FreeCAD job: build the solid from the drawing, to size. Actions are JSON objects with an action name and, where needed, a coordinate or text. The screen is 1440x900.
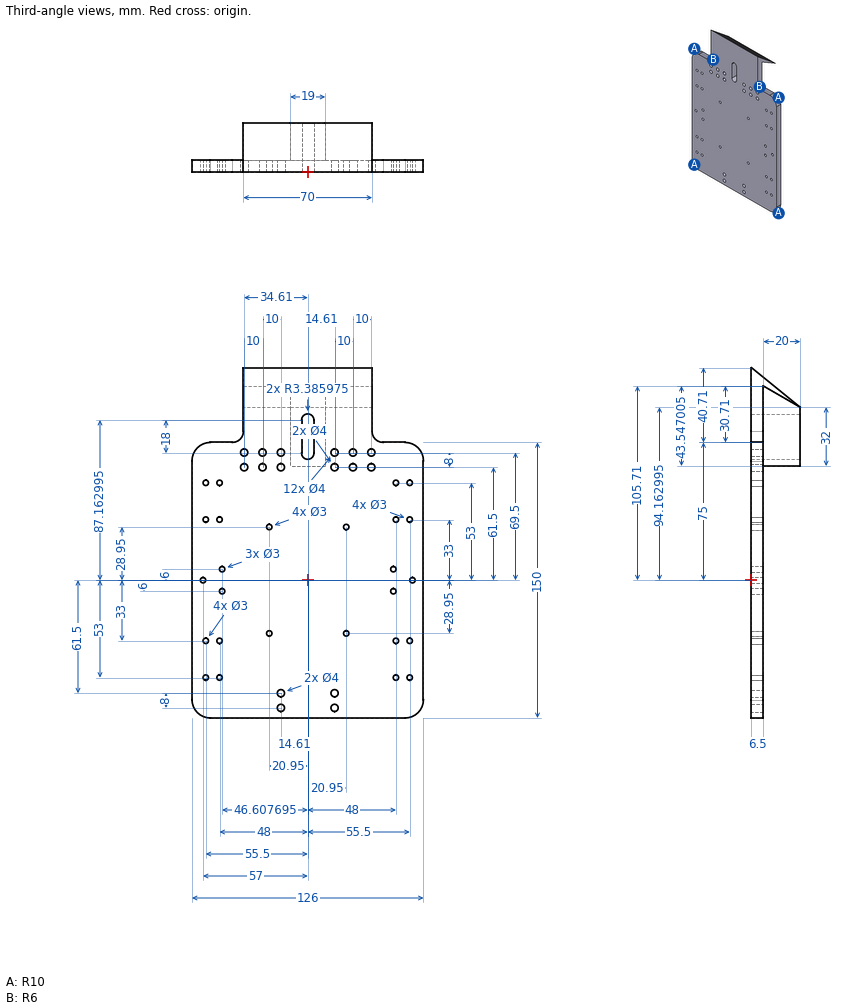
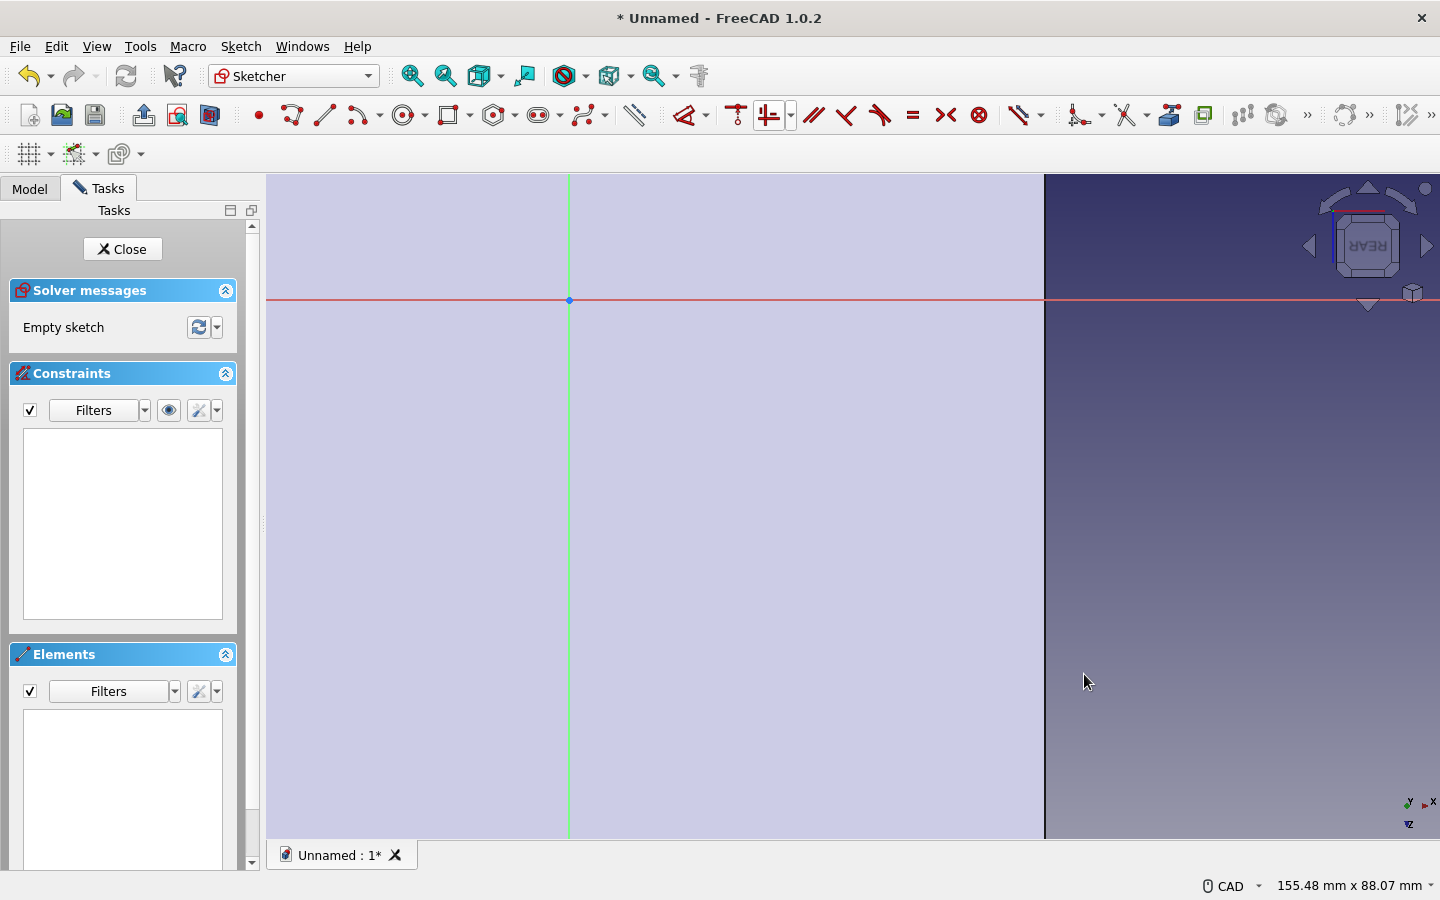
{"action": "key", "text": "g c"}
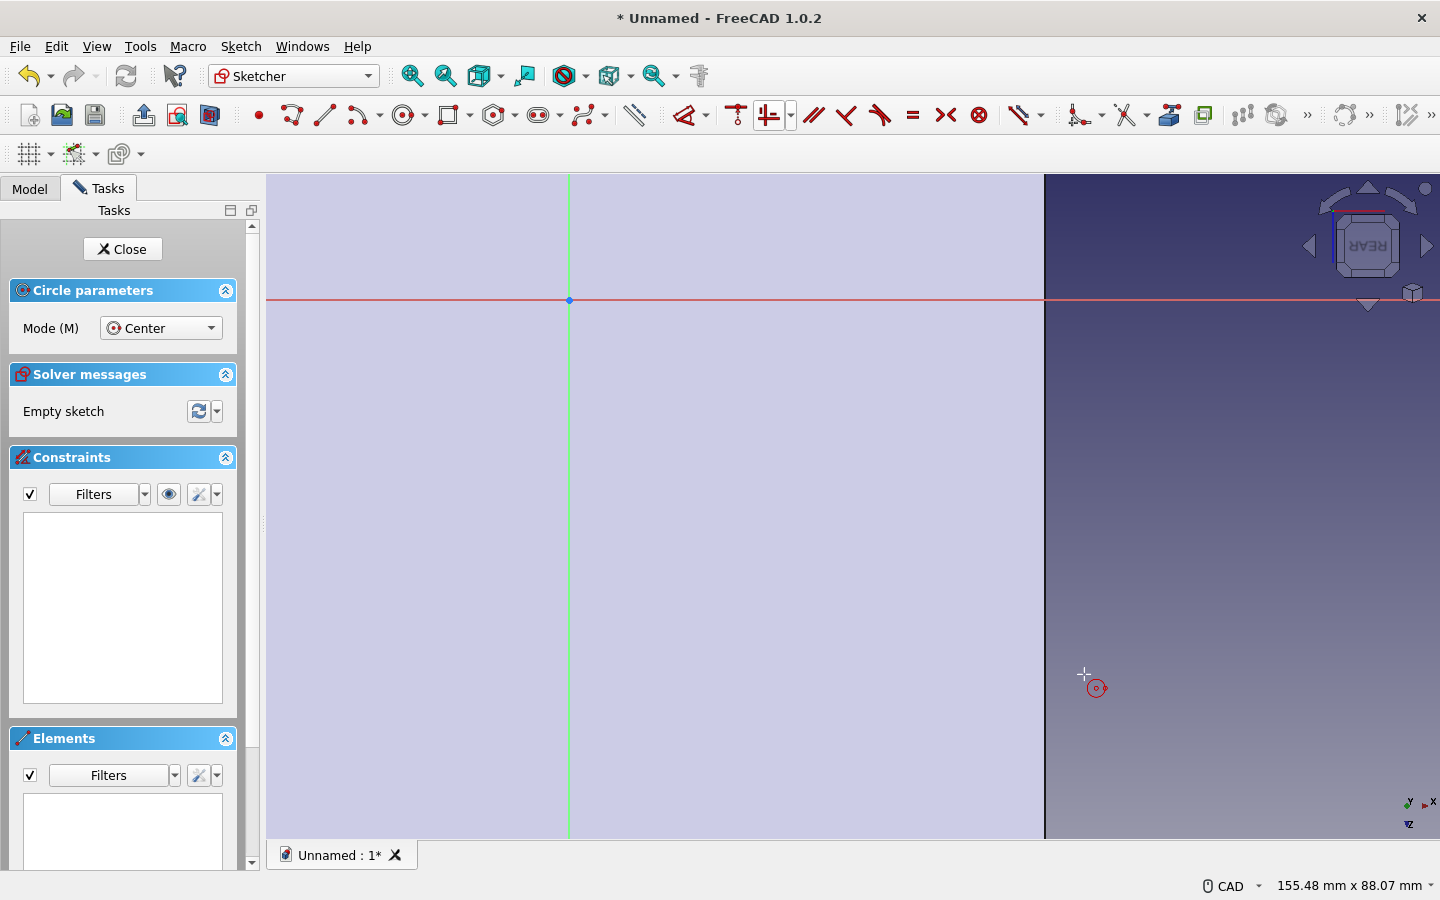
{"action": "scroll", "coordinate": [988, 549], "scroll_direction": "up", "scroll_amount": 4}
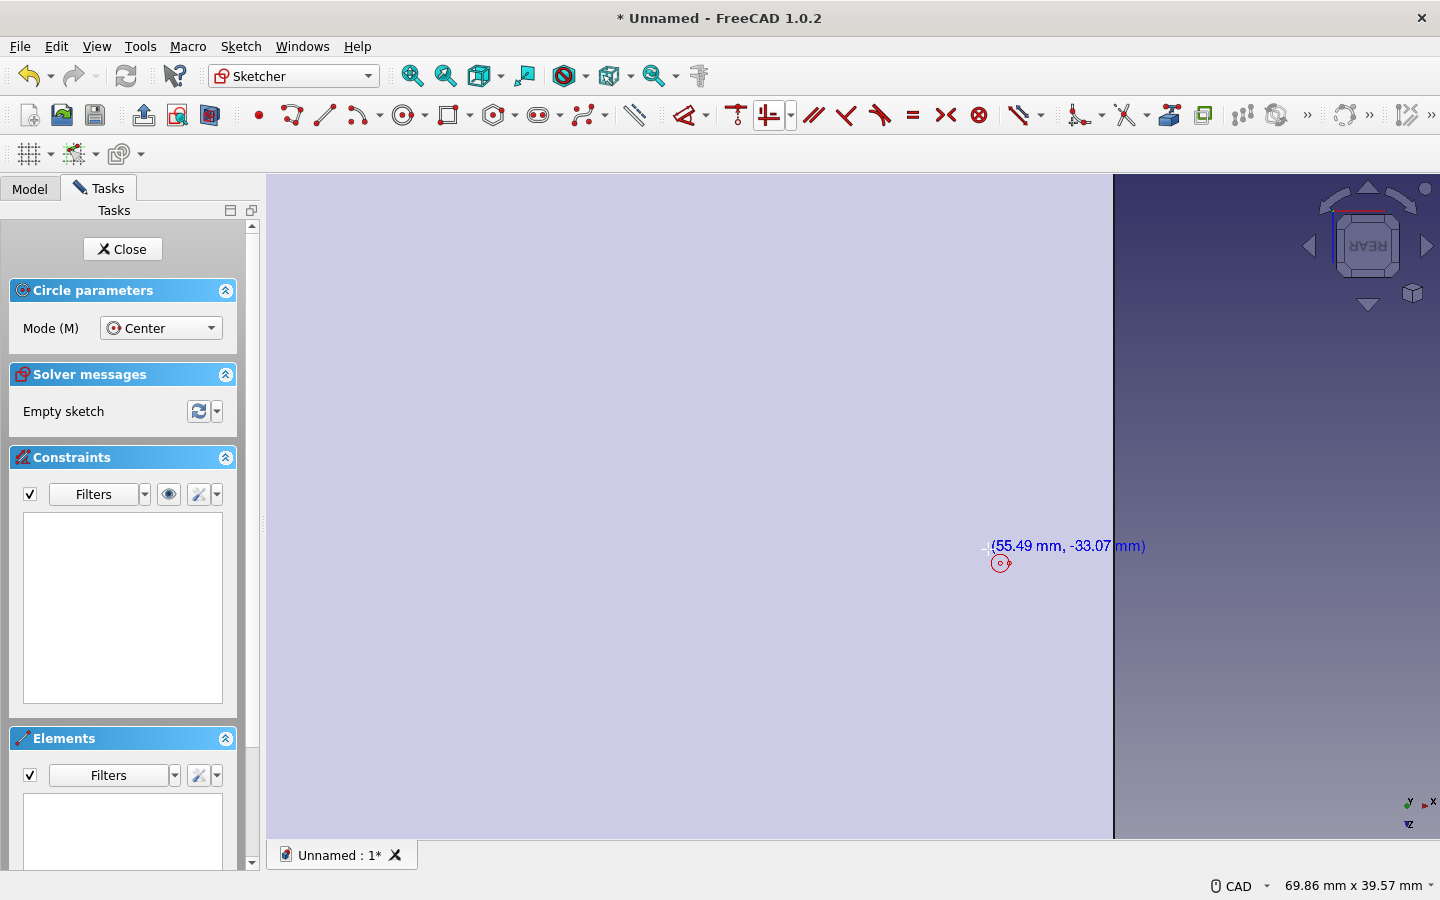
{"action": "left_click", "coordinate": [987, 549]}
{"action": "mouse_move", "coordinate": [1005, 532]}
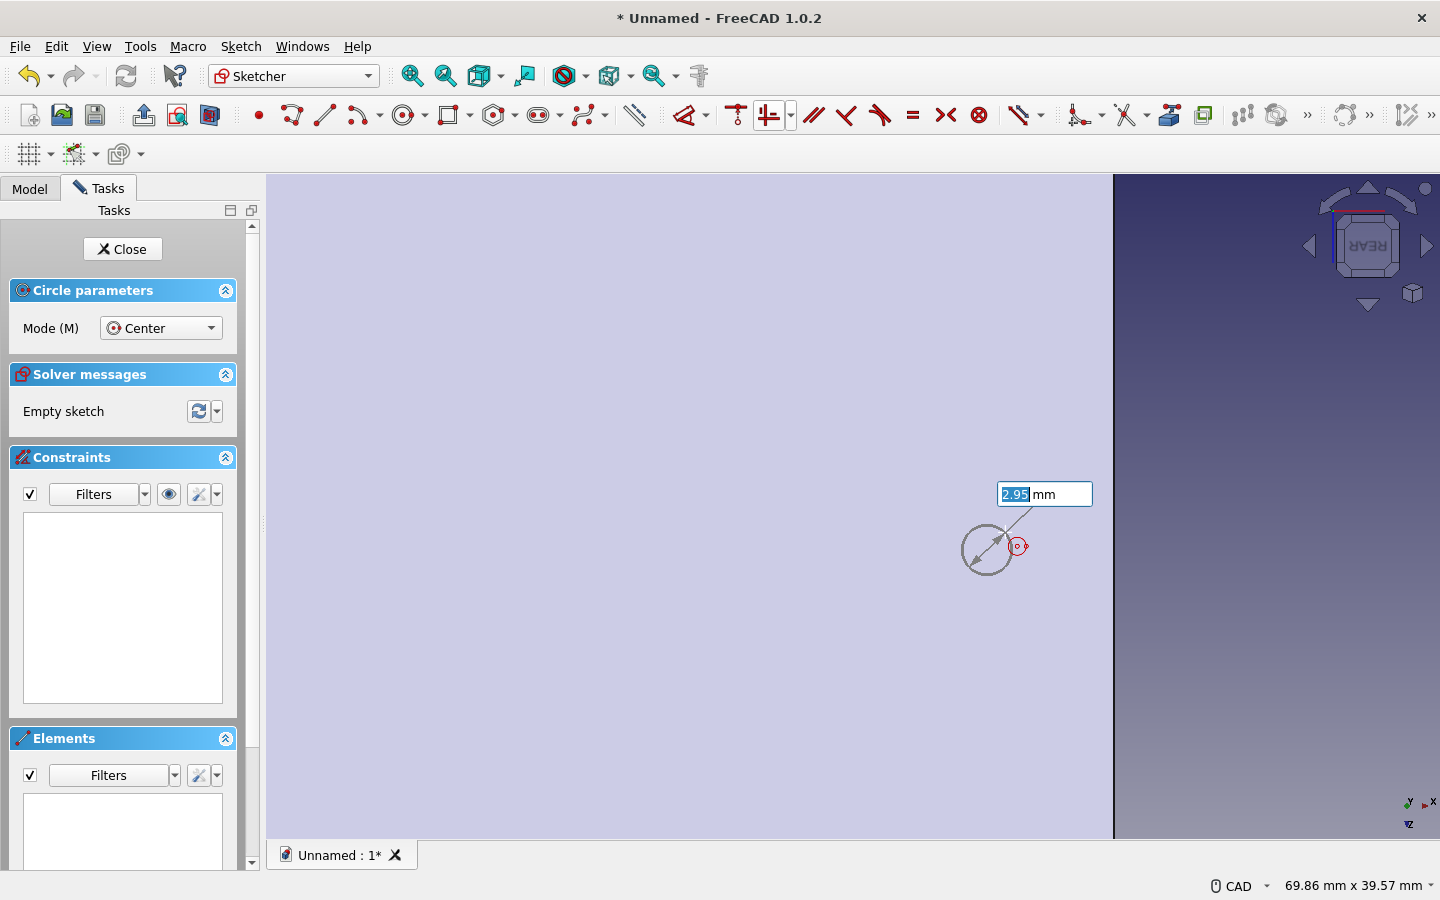
{"action": "type", "text": "3"}
{"action": "key", "text": "Return"}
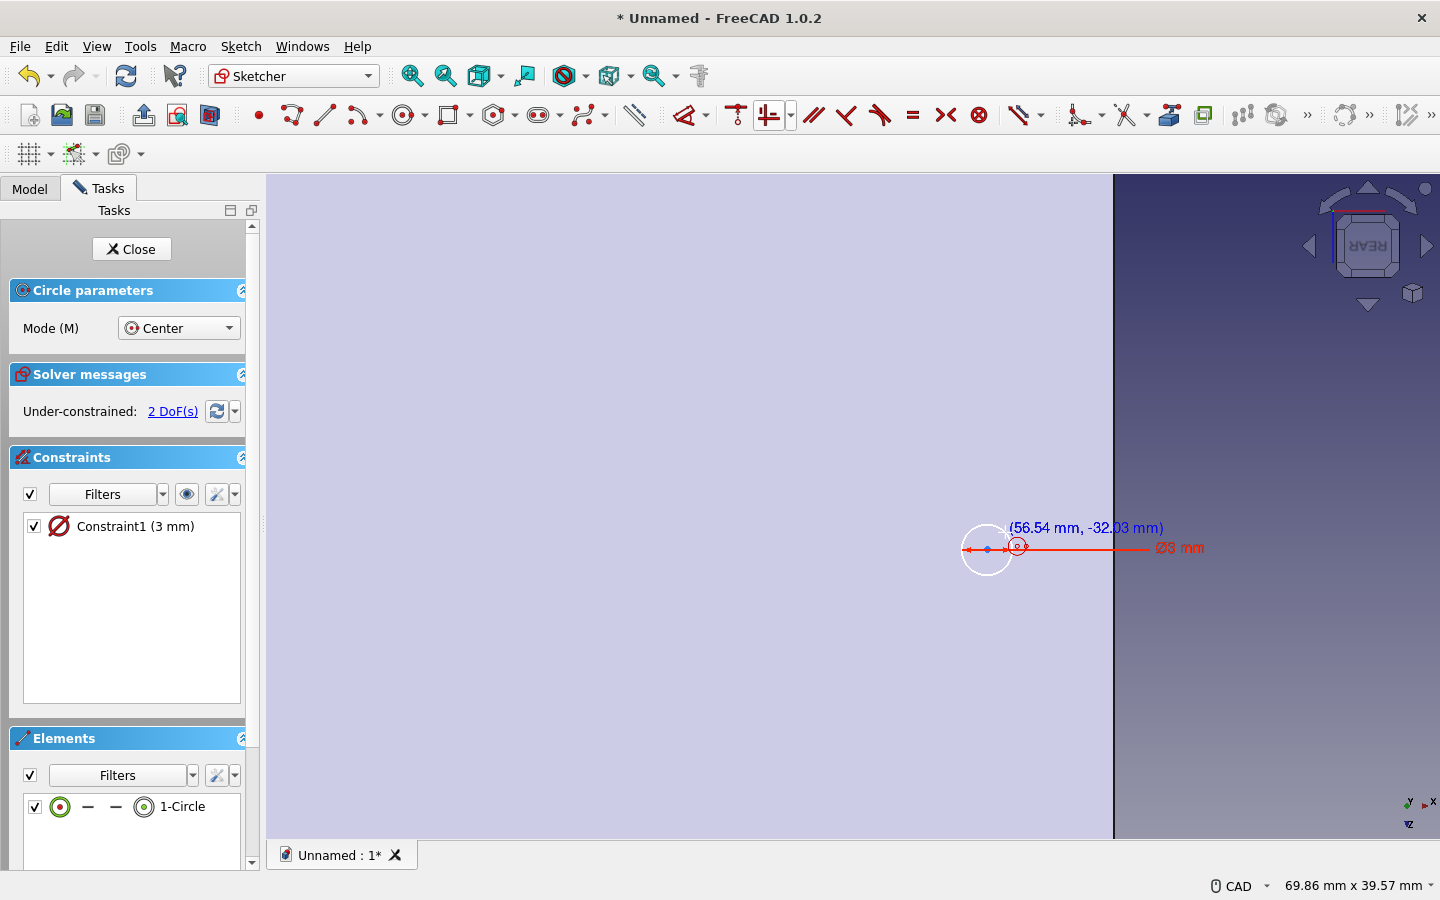
{"action": "left_click", "coordinate": [861, 549]}
{"action": "mouse_move", "coordinate": [879, 532]}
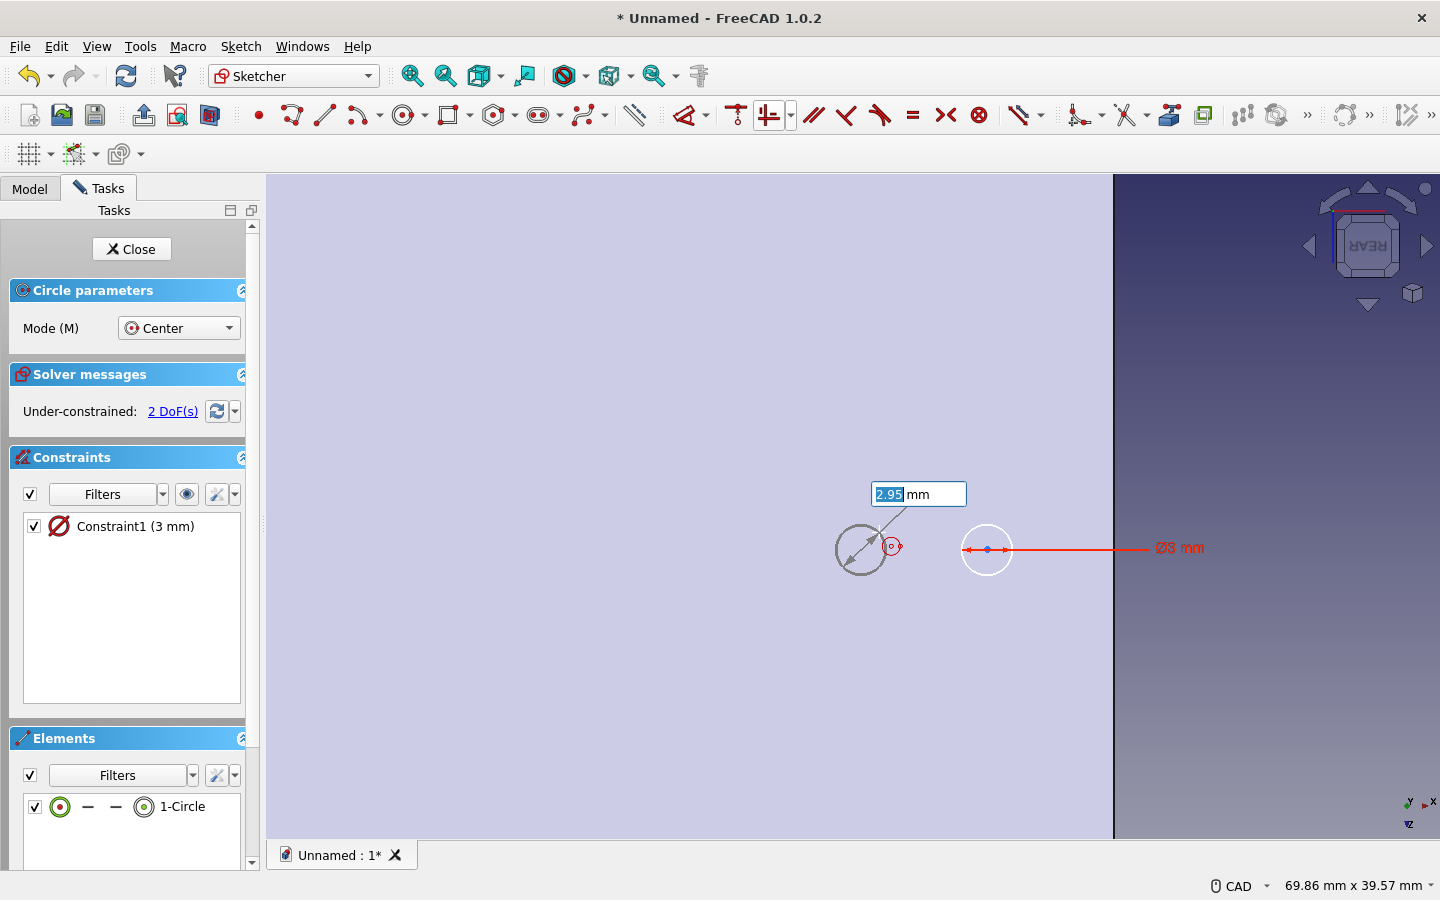
{"action": "type", "text": "3"}
{"action": "key", "text": "Return"}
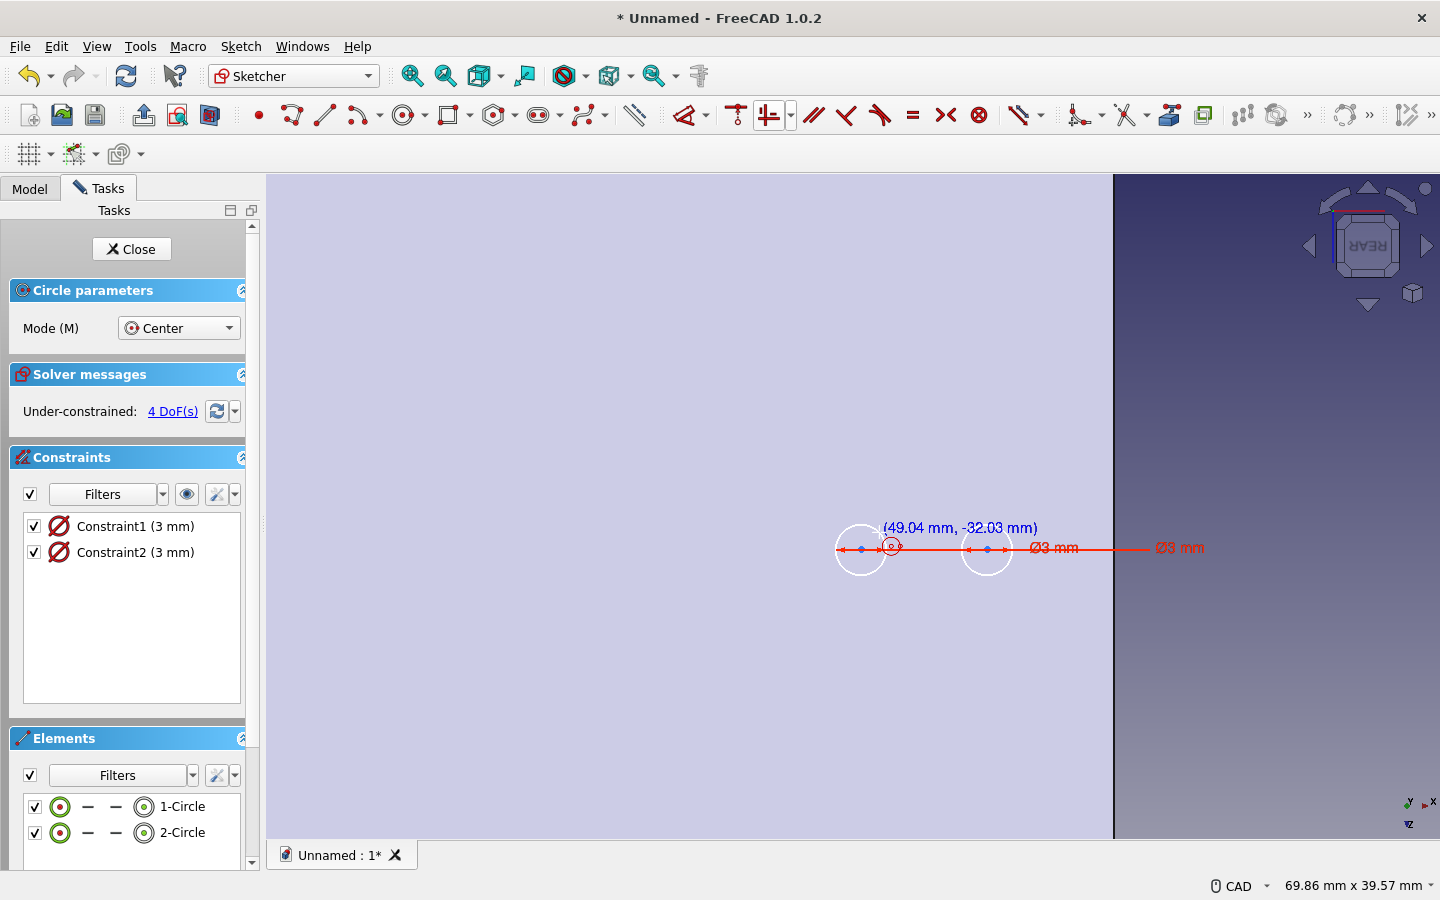
{"action": "scroll", "coordinate": [989, 550], "scroll_direction": "down", "scroll_amount": 4}